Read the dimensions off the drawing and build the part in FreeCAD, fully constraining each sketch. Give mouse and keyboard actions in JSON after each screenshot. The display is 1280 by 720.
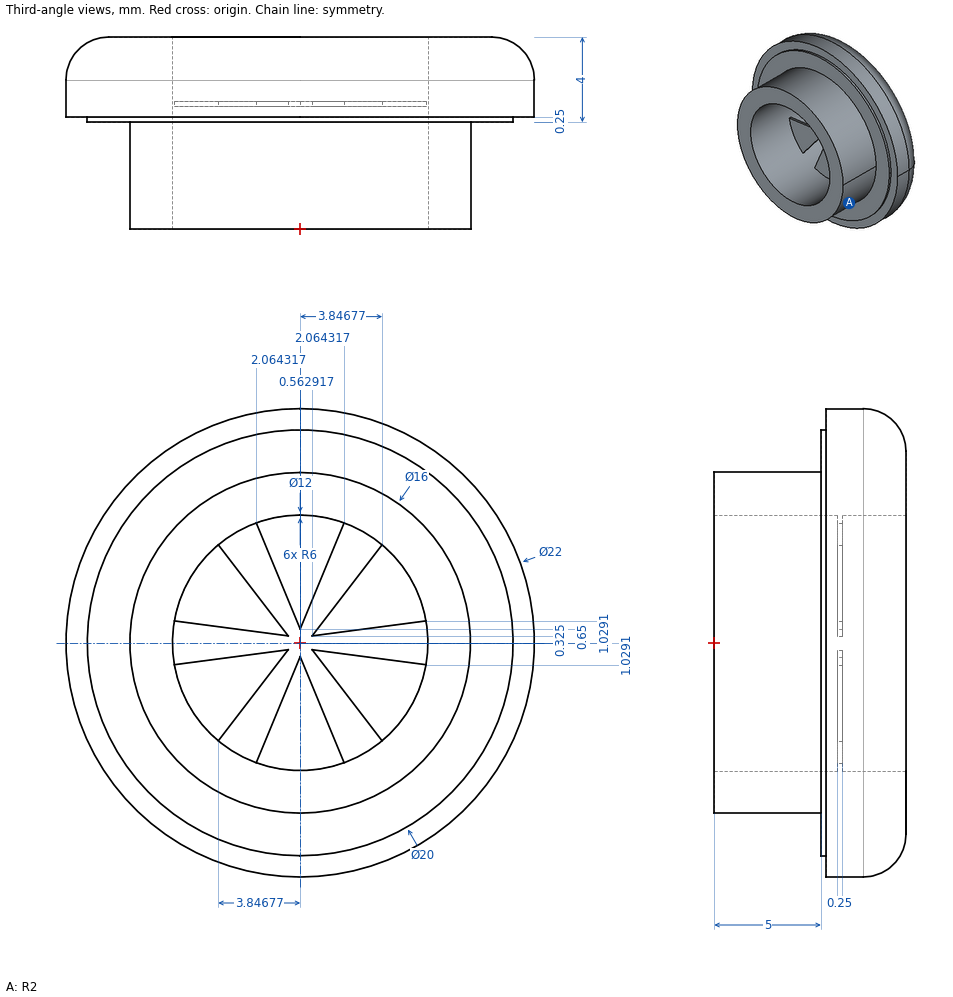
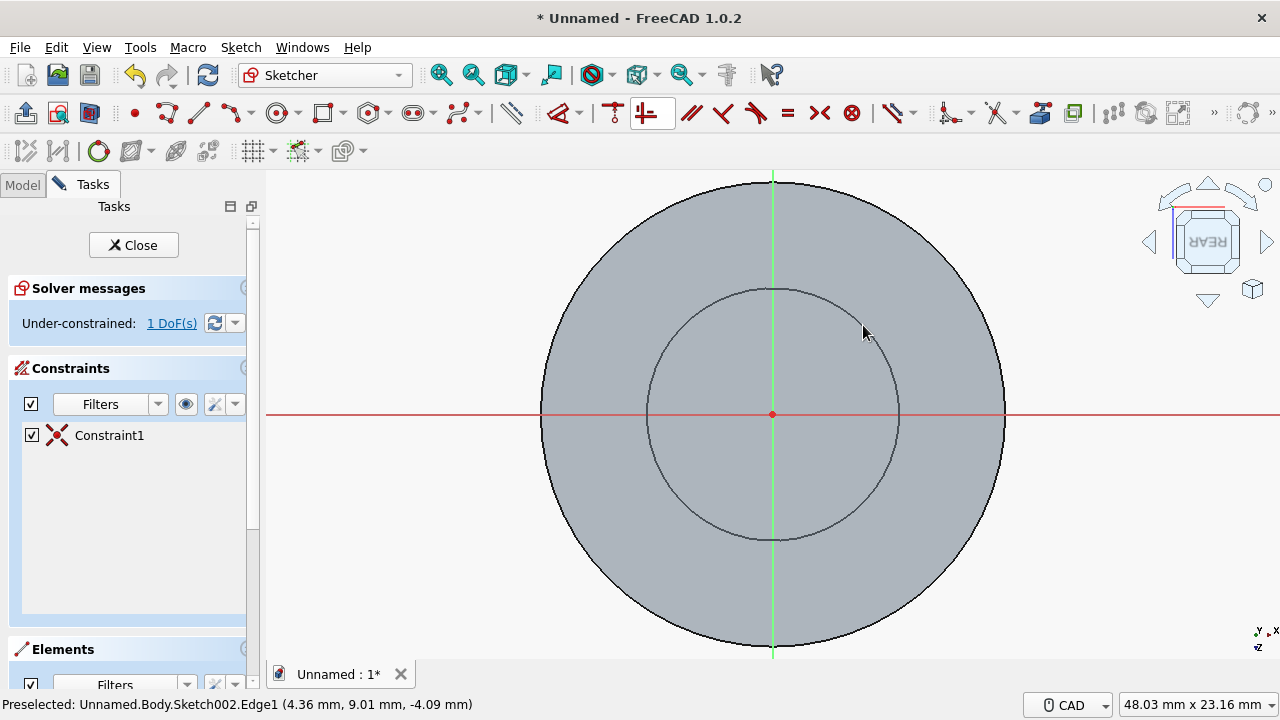
{"action": "key", "text": "d"}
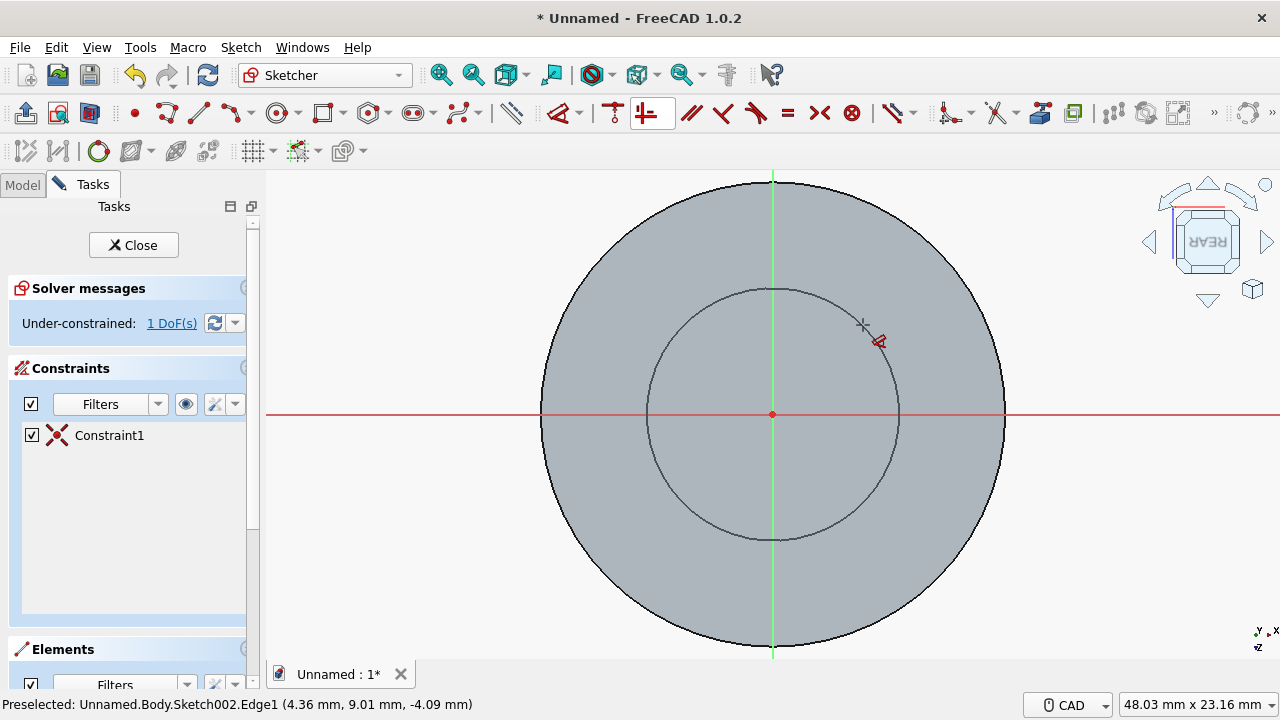
{"action": "left_click", "coordinate": [862, 325]}
{"action": "left_click", "coordinate": [885, 302]}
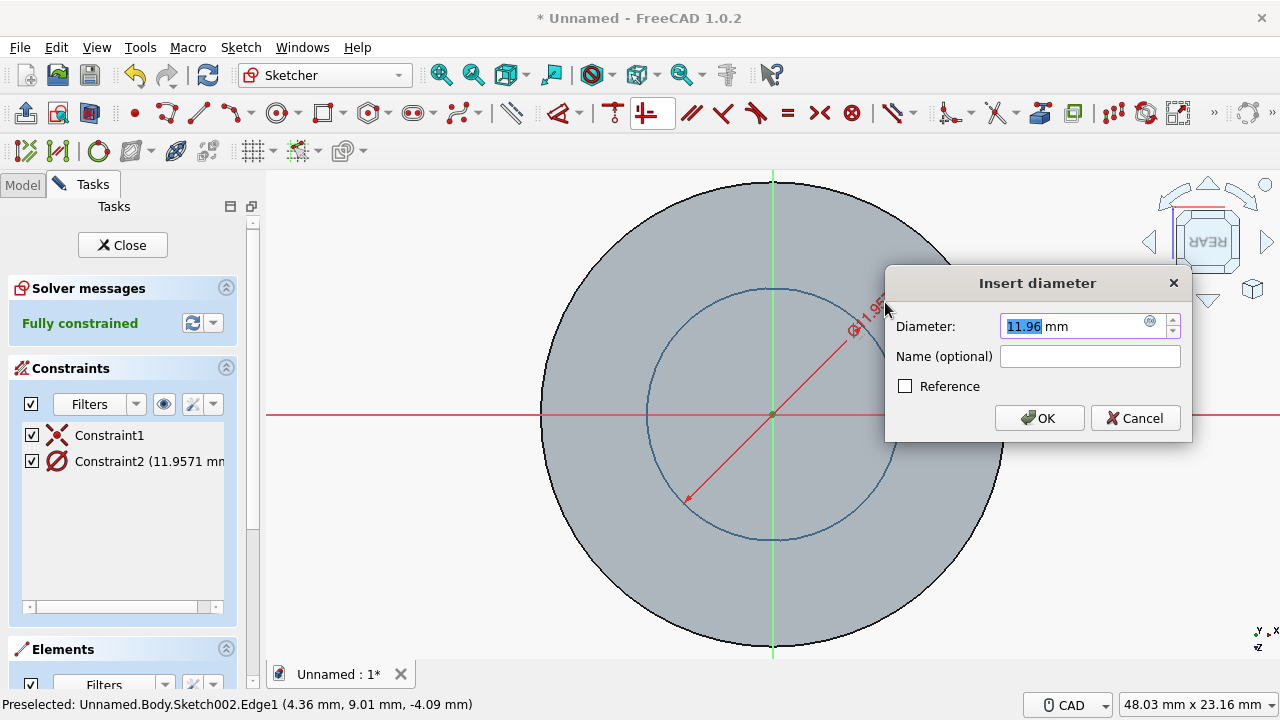
{"action": "type", "text": "12"}
{"action": "key", "text": "Return"}
{"action": "key", "text": "Escape"}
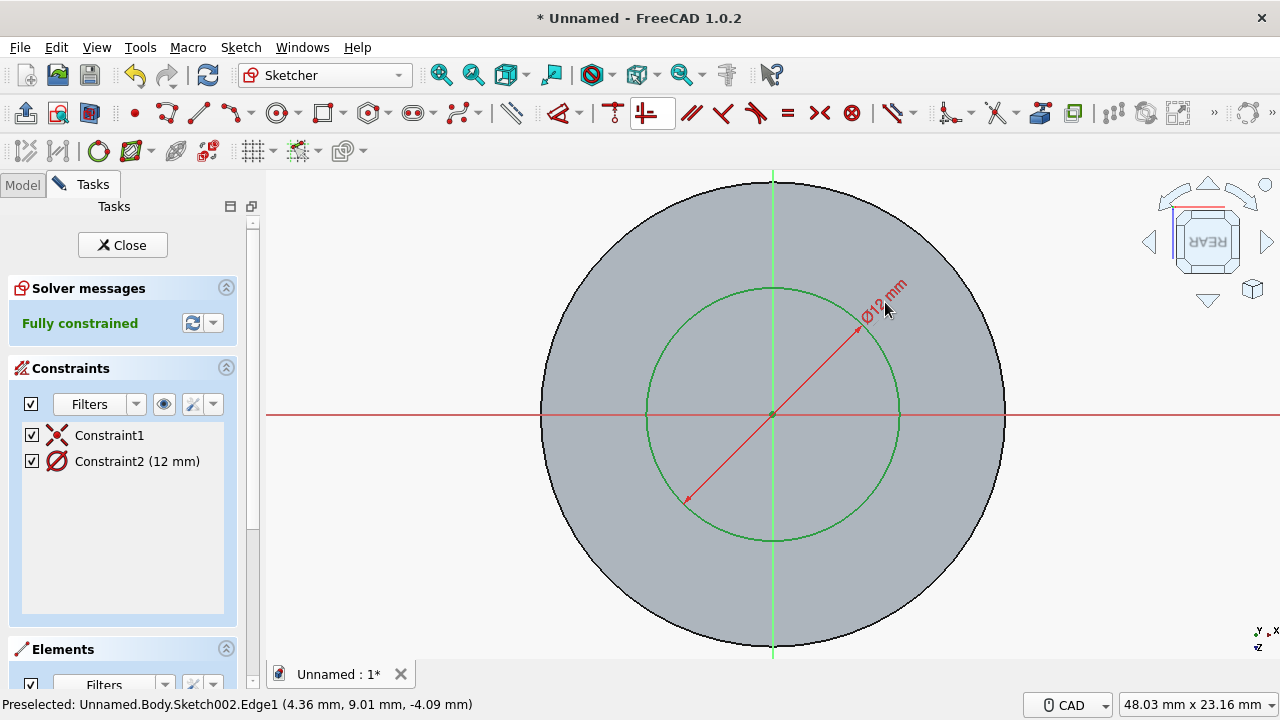
{"action": "left_click", "coordinate": [123, 245]}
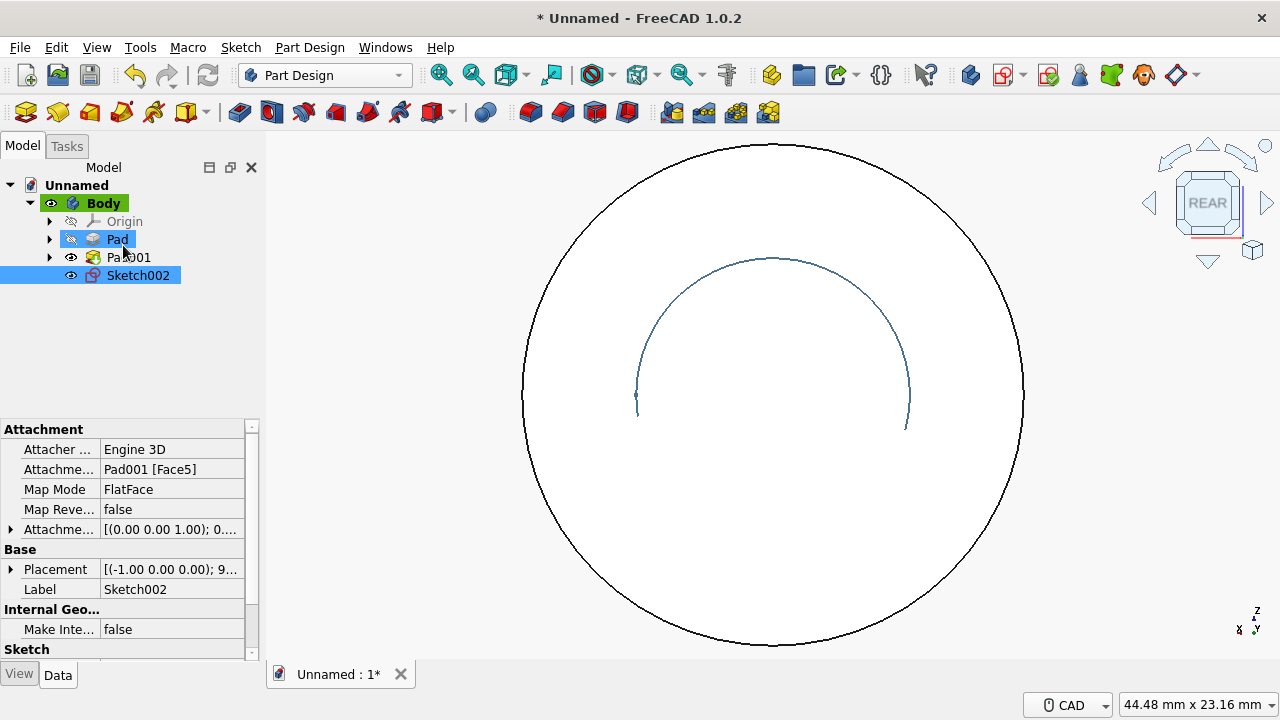
{"action": "left_click", "coordinate": [240, 112]}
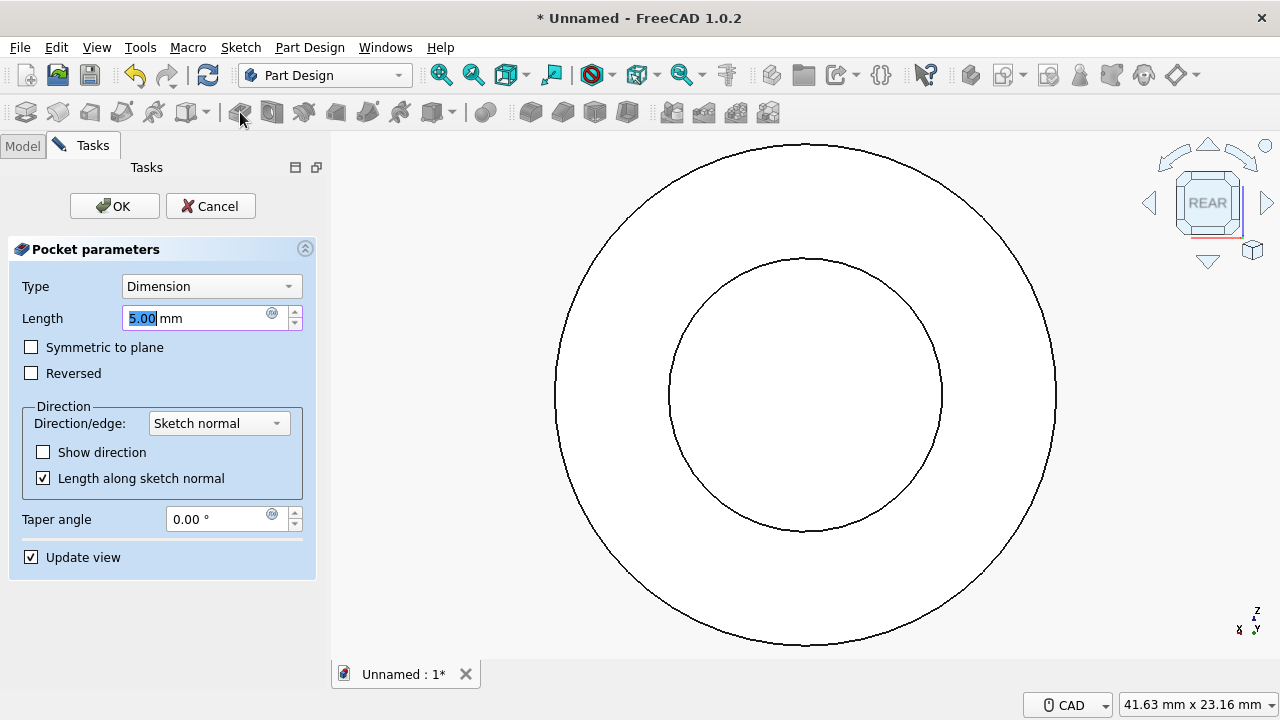
{"action": "left_click", "coordinate": [212, 286]}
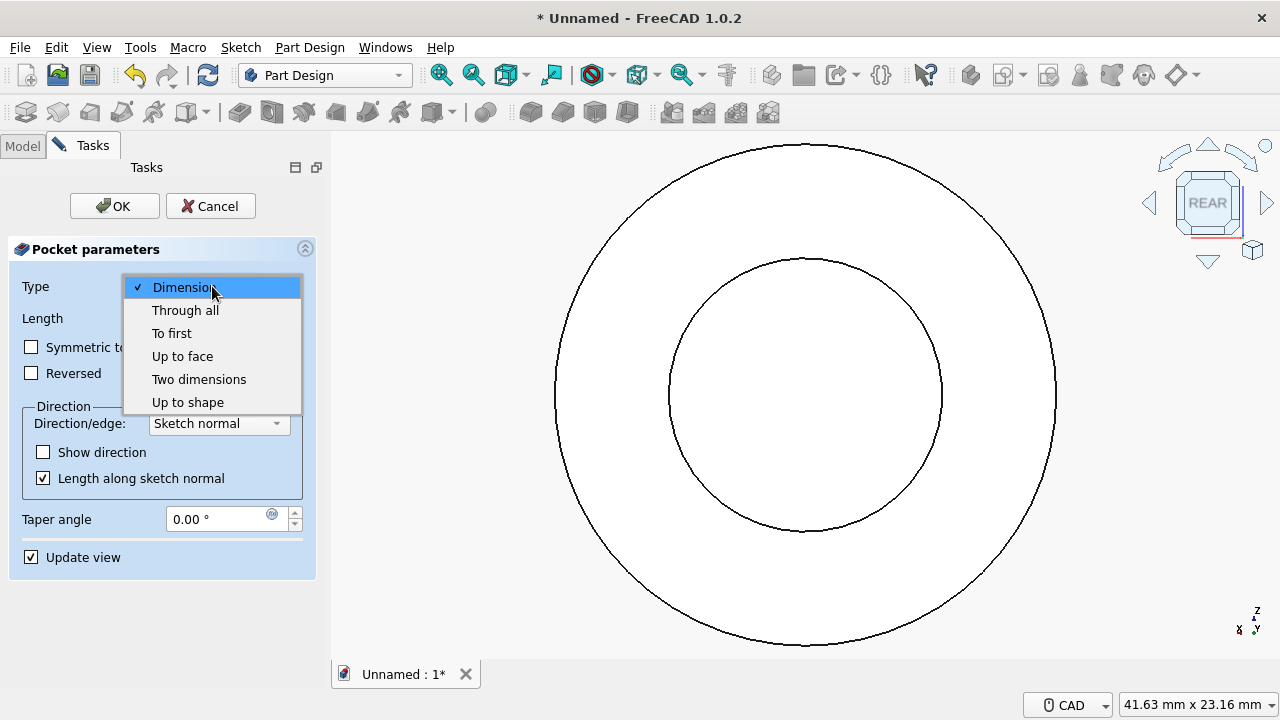
{"action": "left_click", "coordinate": [212, 334]}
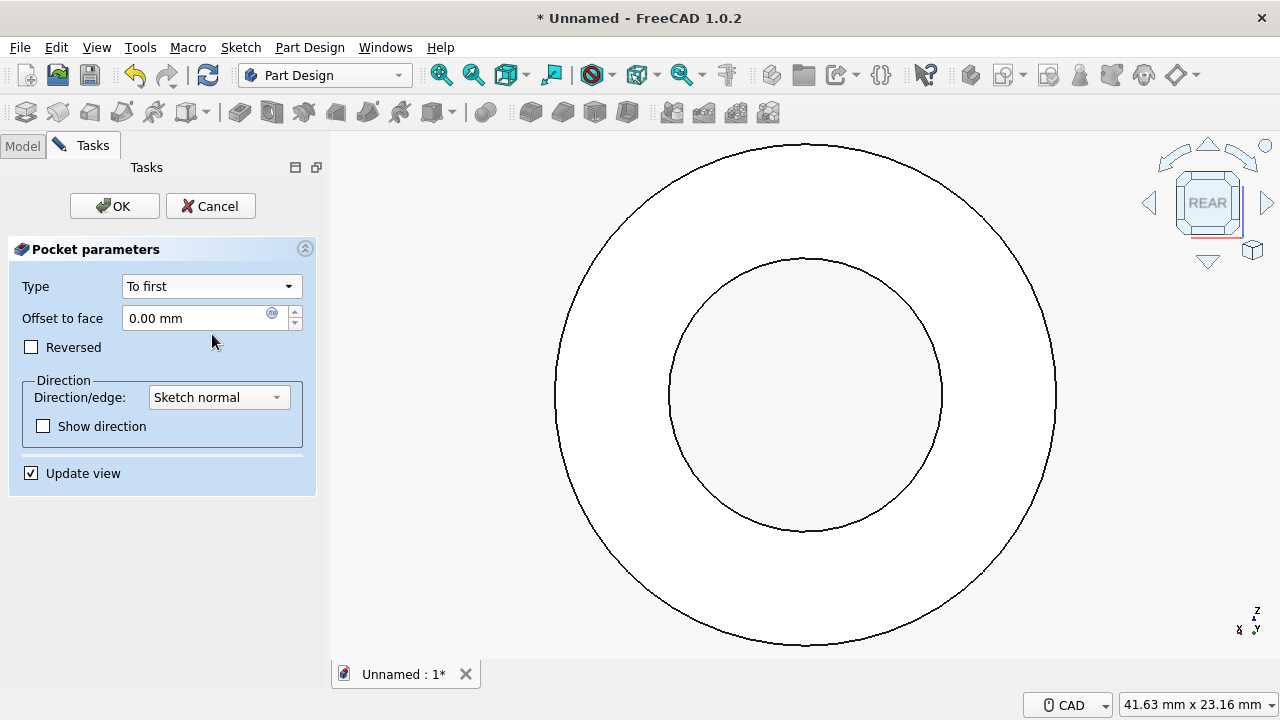
{"action": "left_click", "coordinate": [115, 206]}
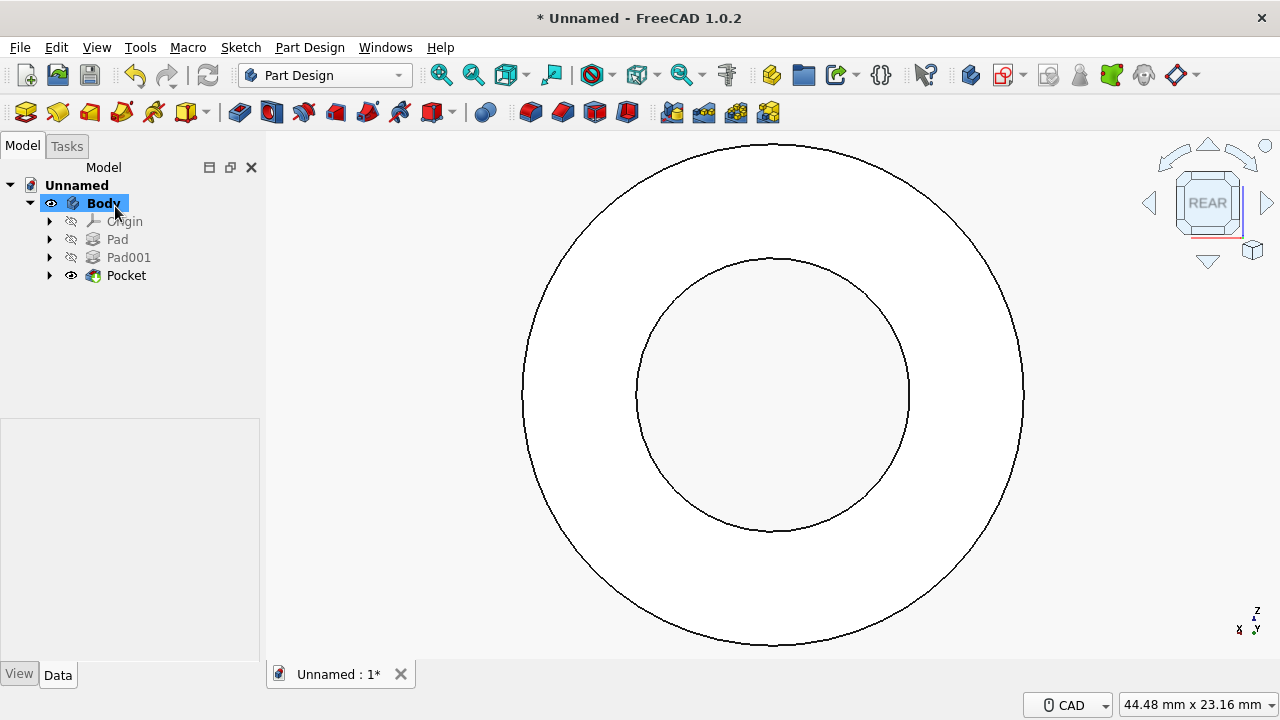
{"action": "left_click", "coordinate": [50, 221]}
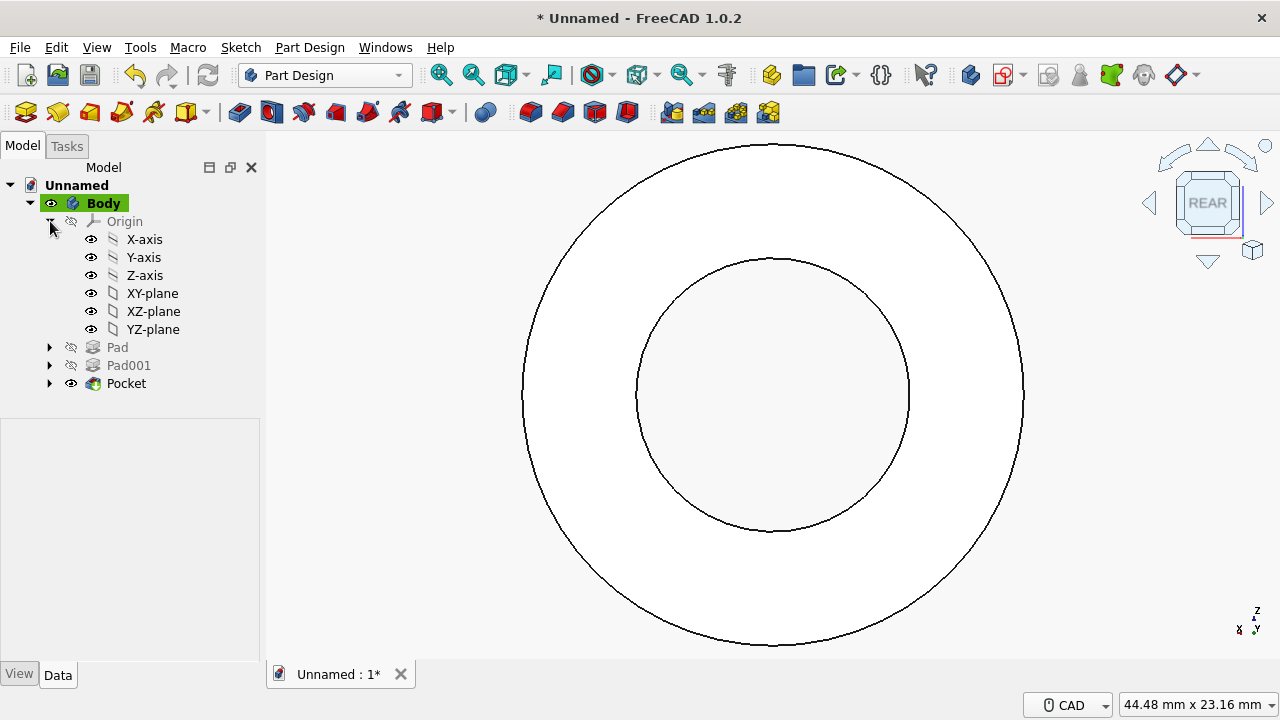
{"action": "left_click", "coordinate": [136, 311]}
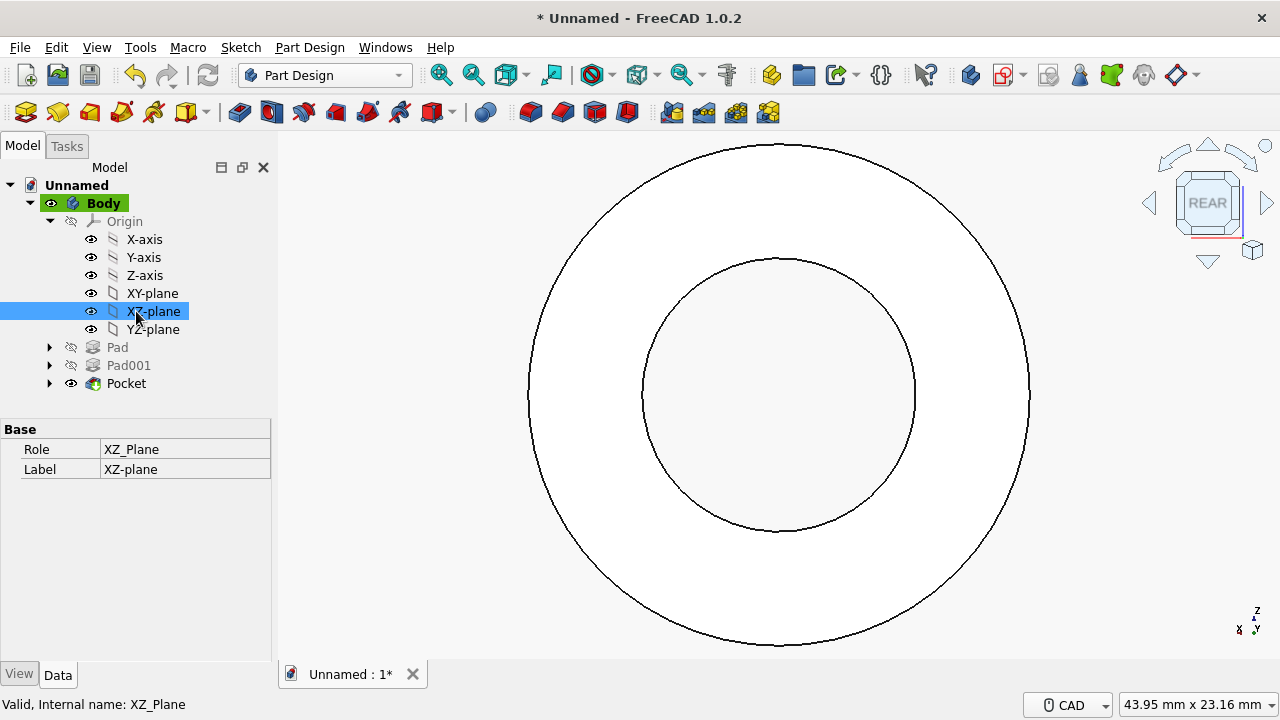
{"action": "left_click", "coordinate": [1176, 76]}